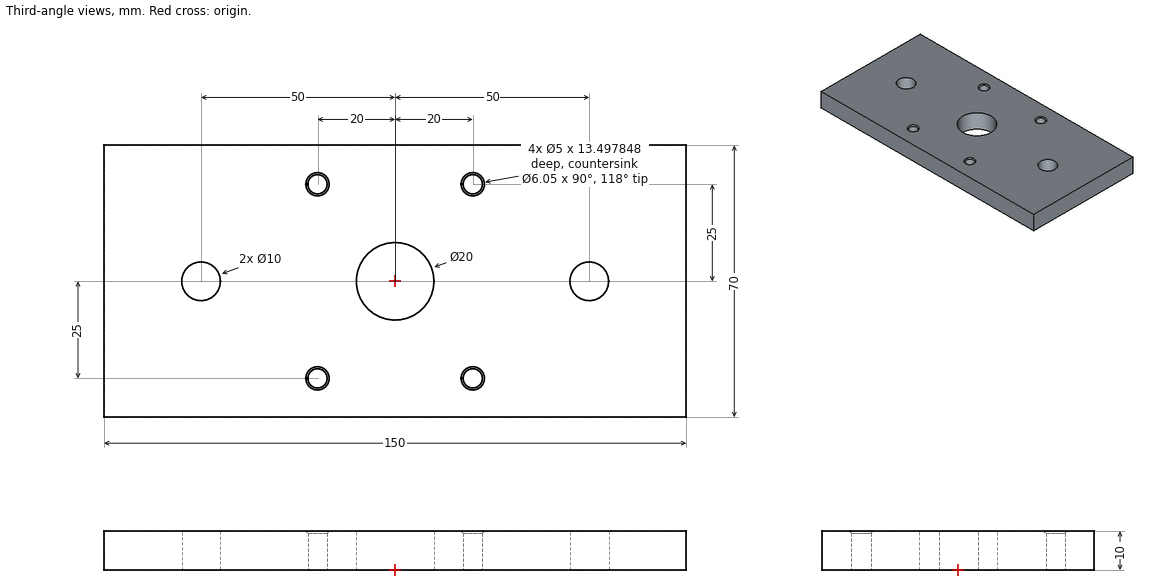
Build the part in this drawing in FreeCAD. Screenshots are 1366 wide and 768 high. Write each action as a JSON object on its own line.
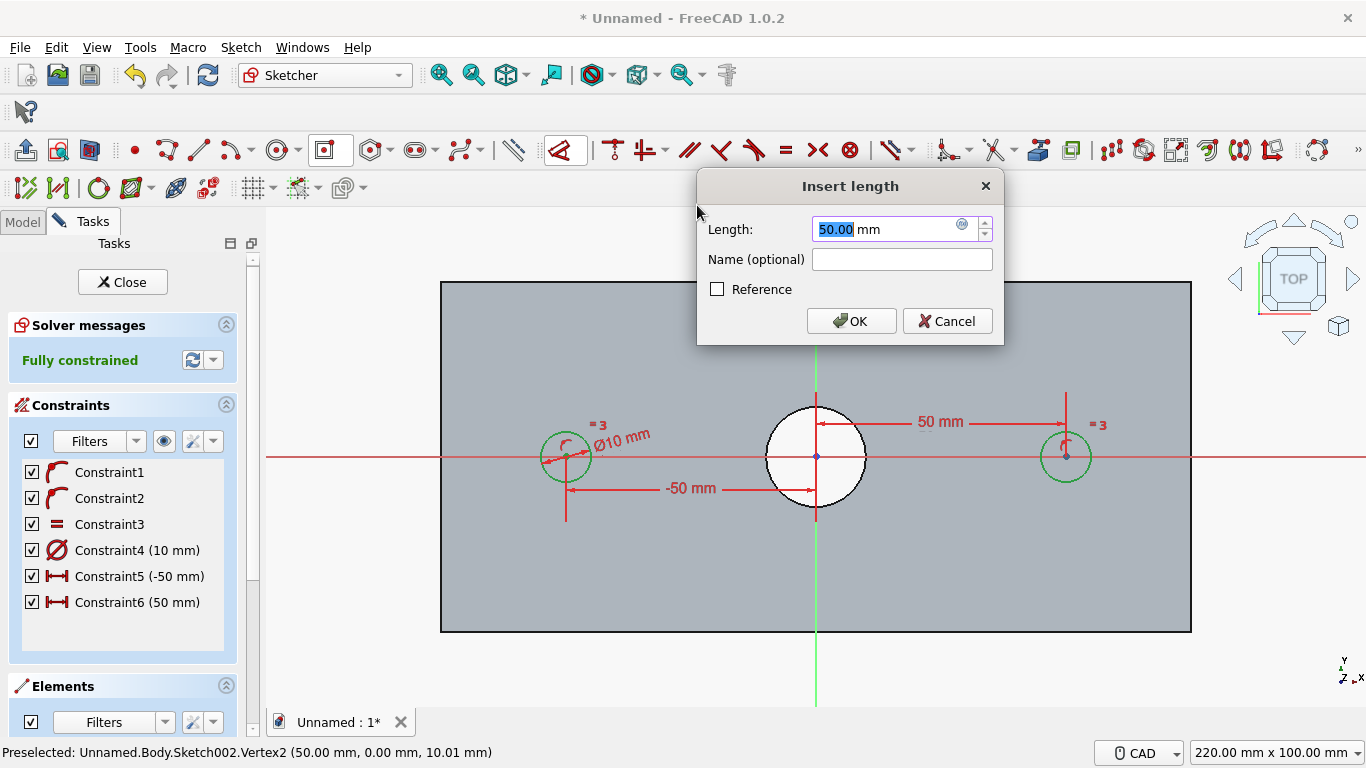
{"action": "type", "text": "50"}
{"action": "key", "text": "Return"}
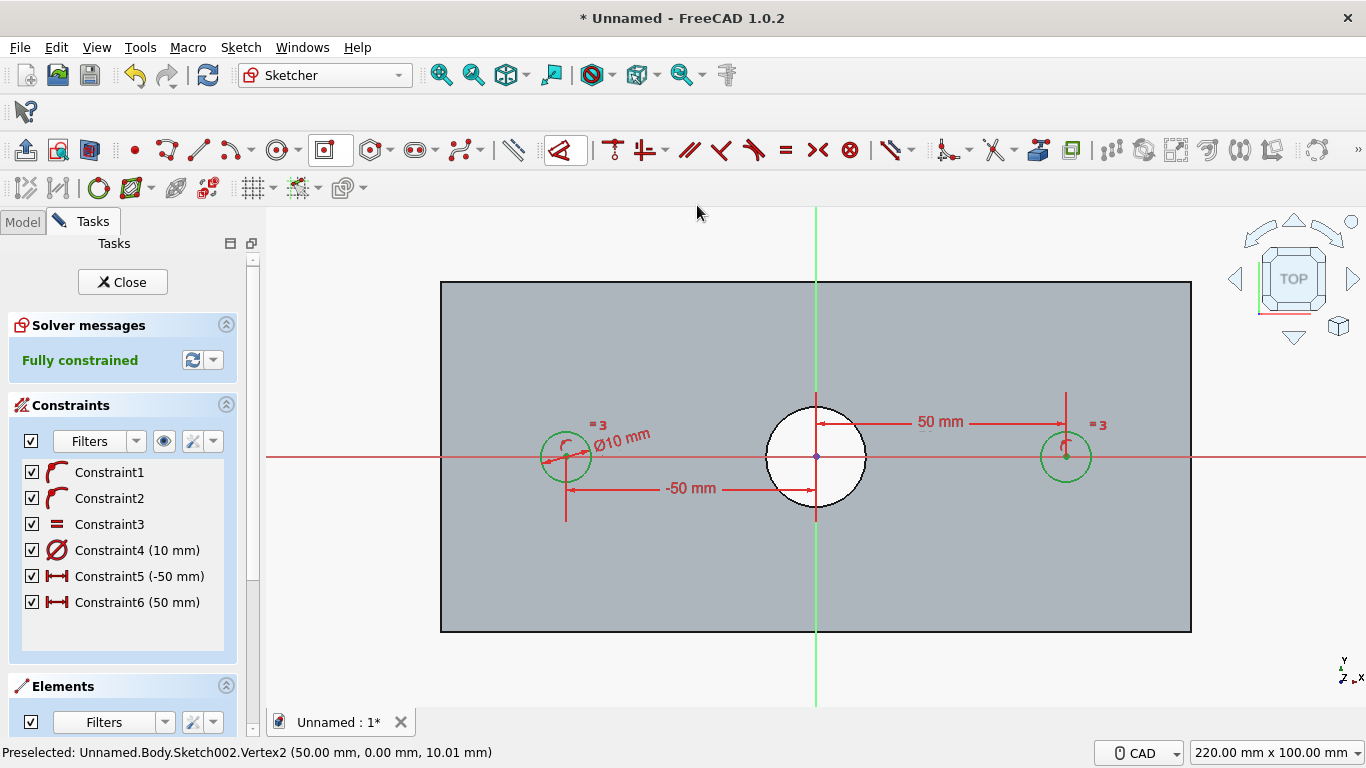
{"action": "left_click", "coordinate": [123, 282]}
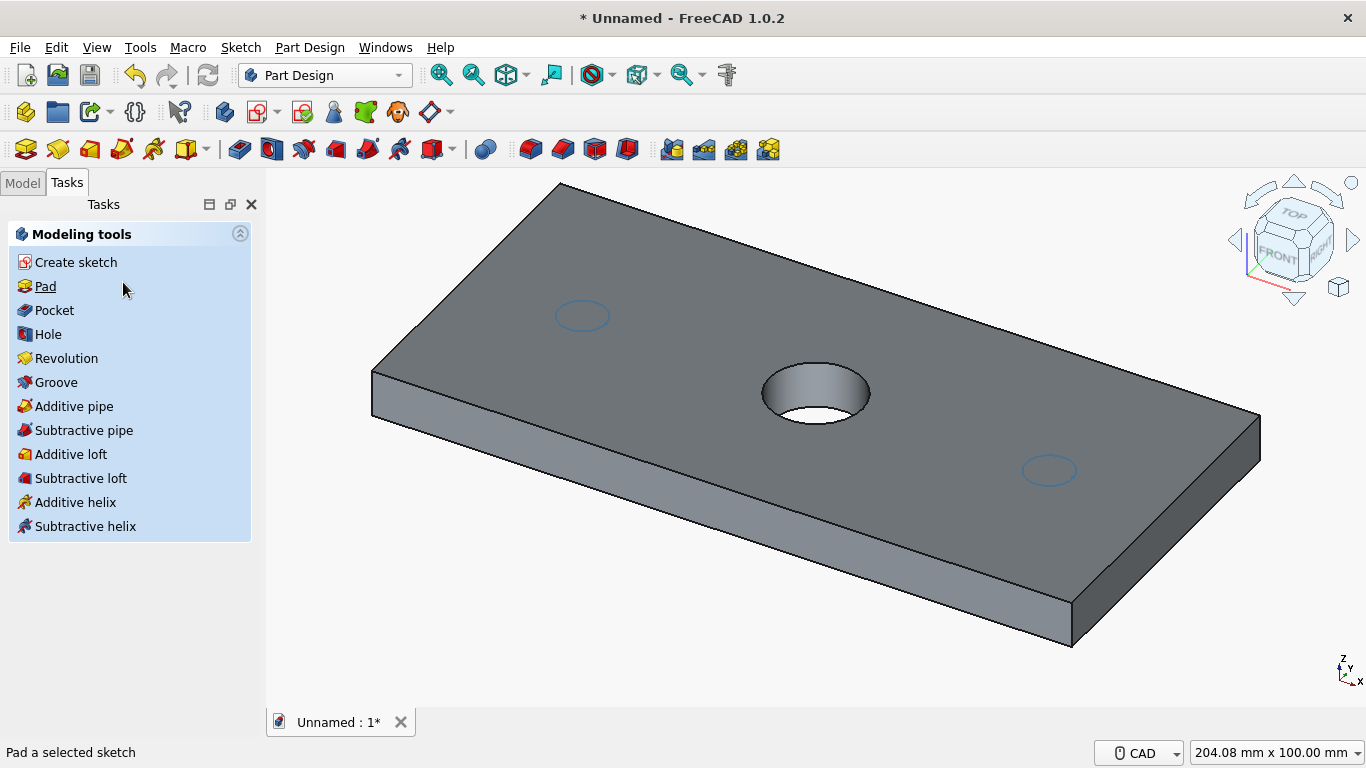
{"action": "left_click", "coordinate": [240, 150]}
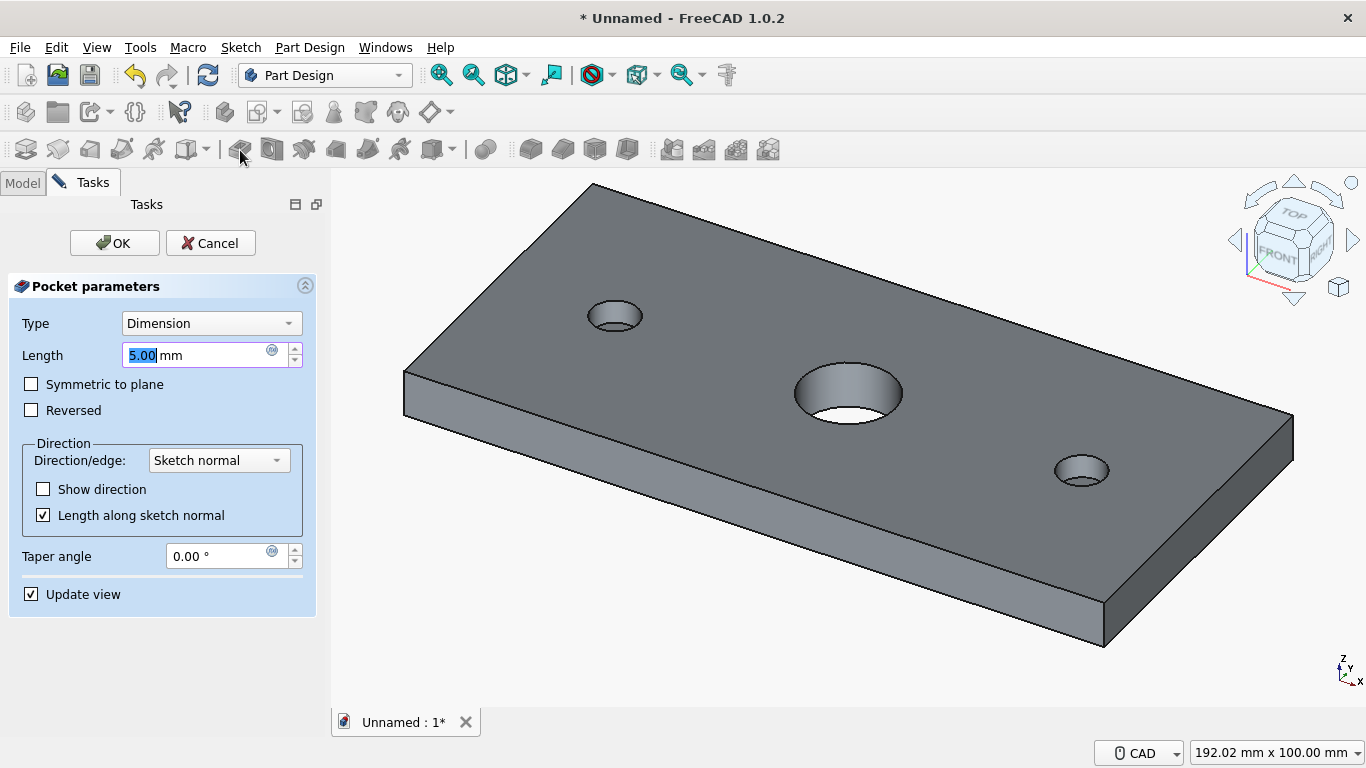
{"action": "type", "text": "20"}
{"action": "key", "text": "Tab"}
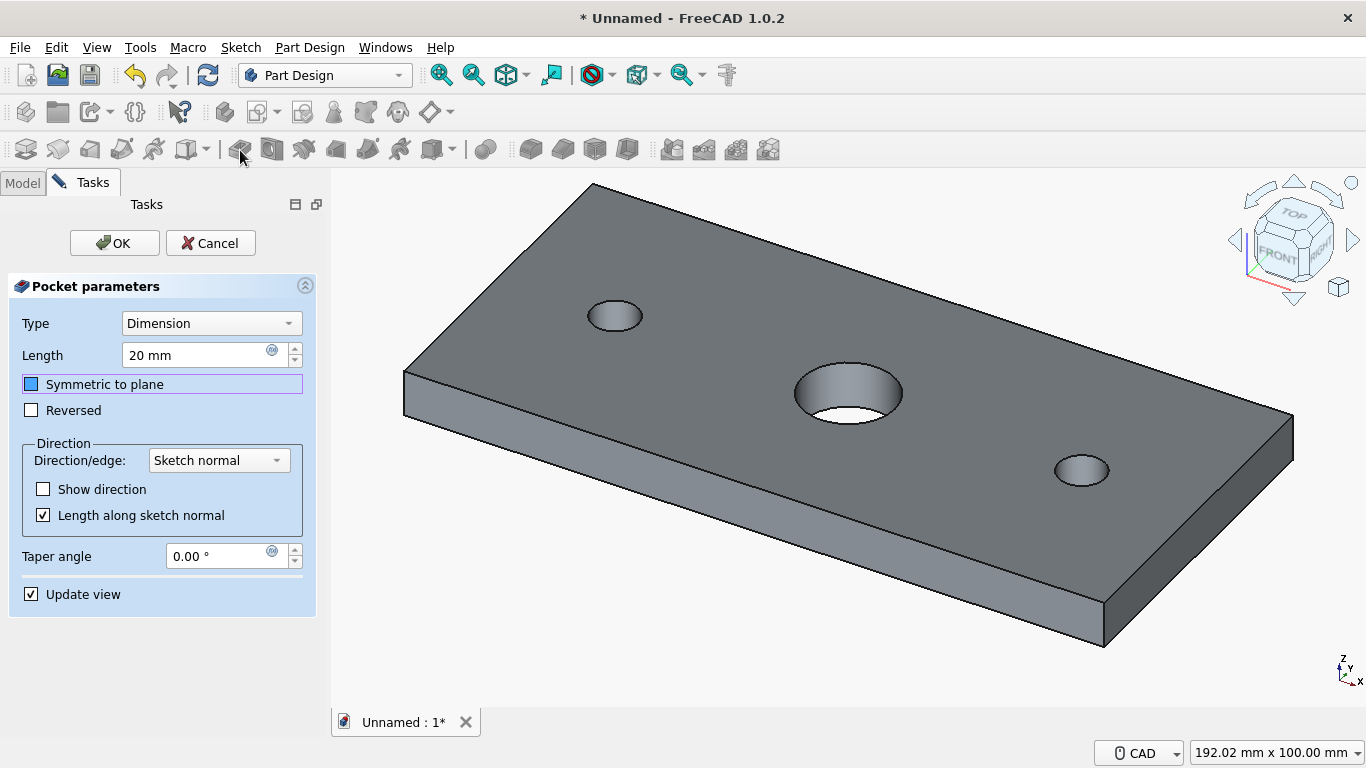
{"action": "left_click", "coordinate": [115, 243]}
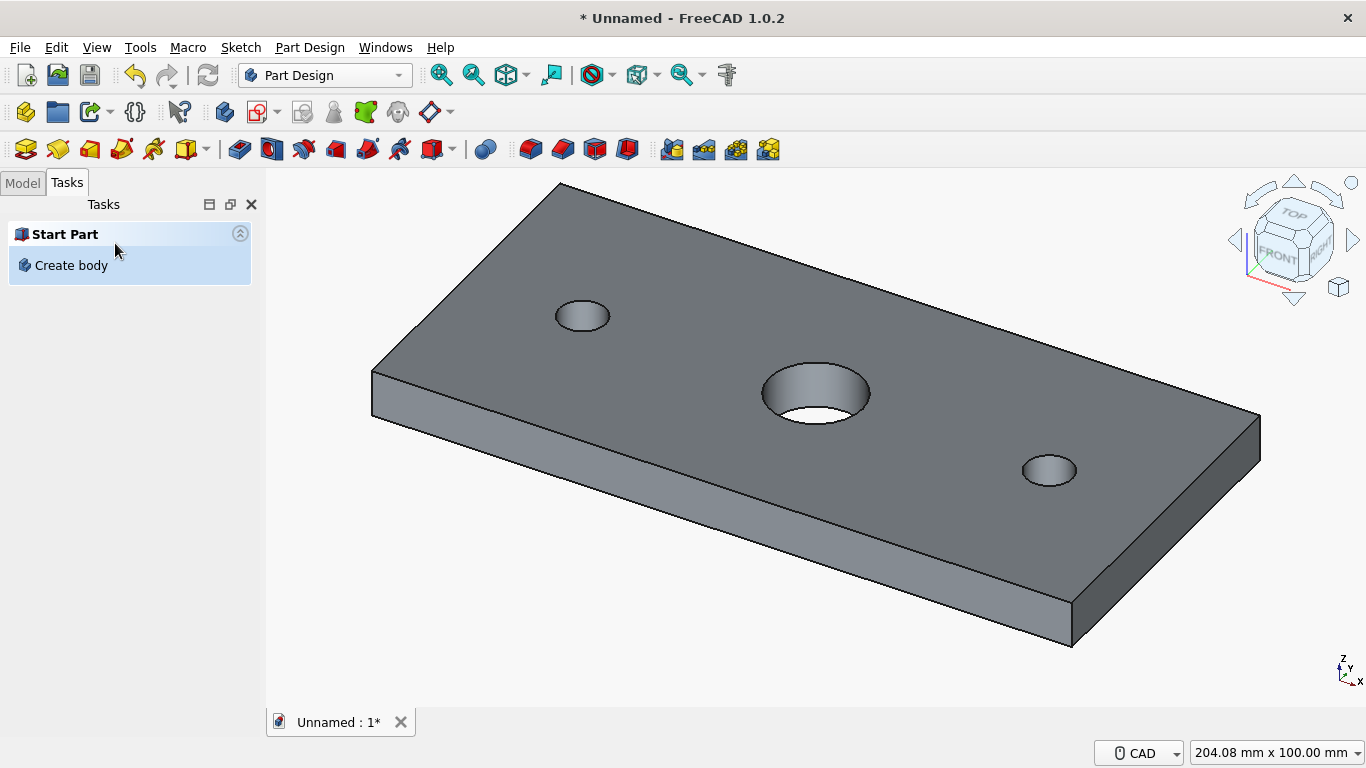
{"action": "left_click", "coordinate": [1070, 405]}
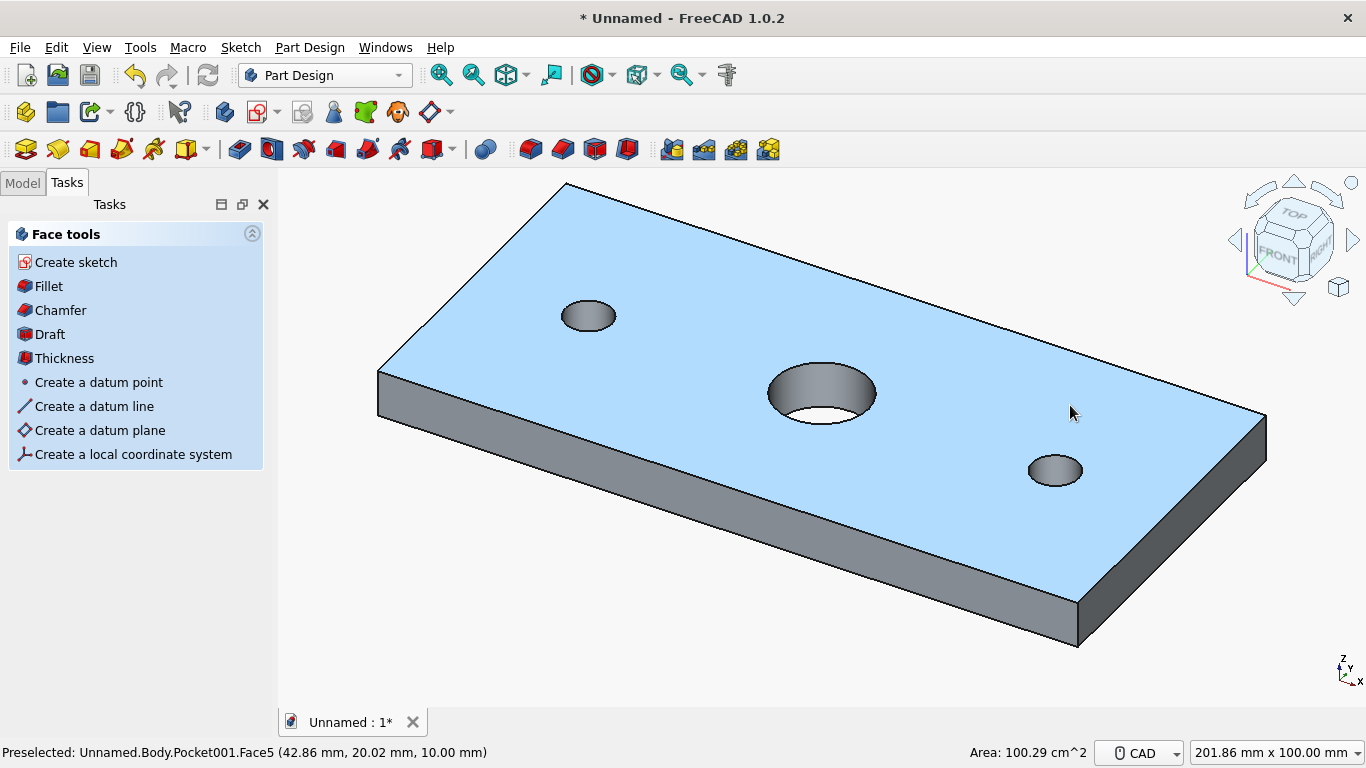
{"action": "left_click", "coordinate": [258, 112]}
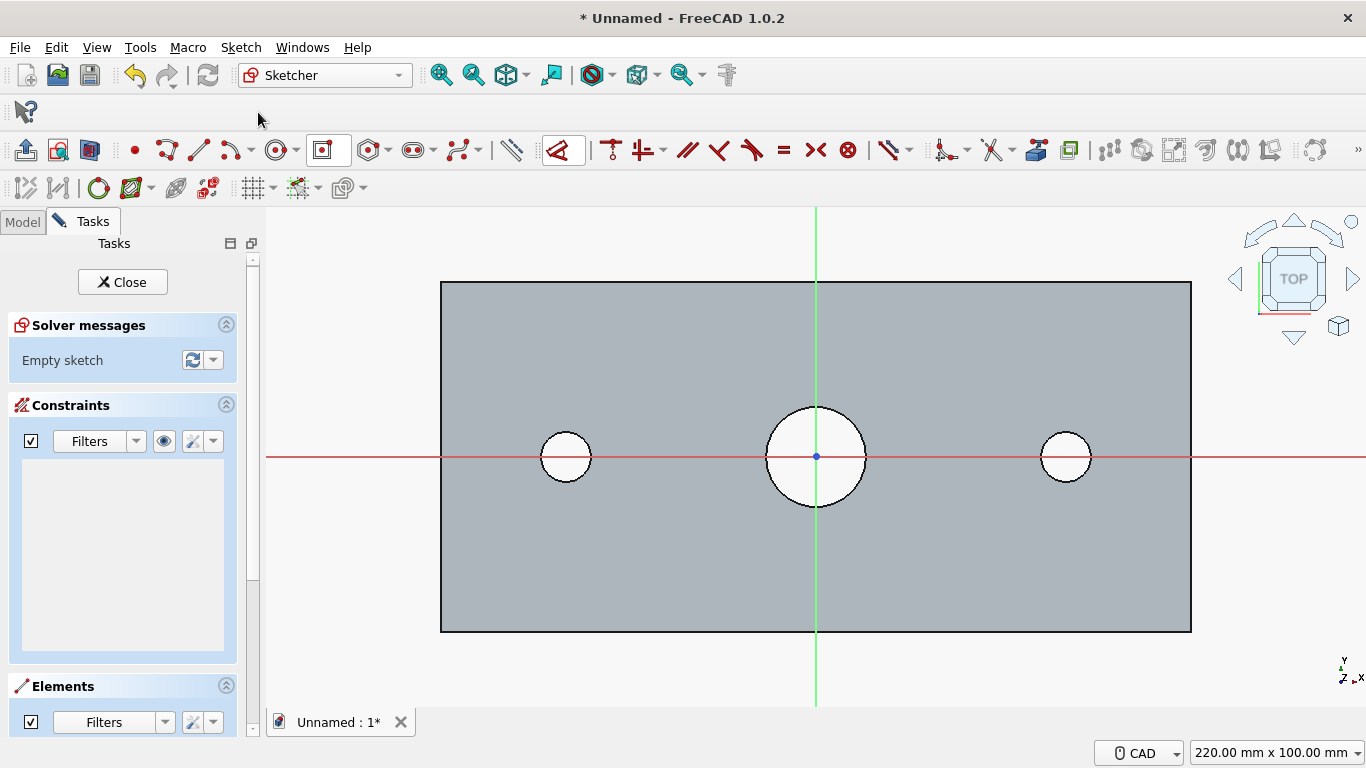
{"action": "left_click", "coordinate": [276, 150]}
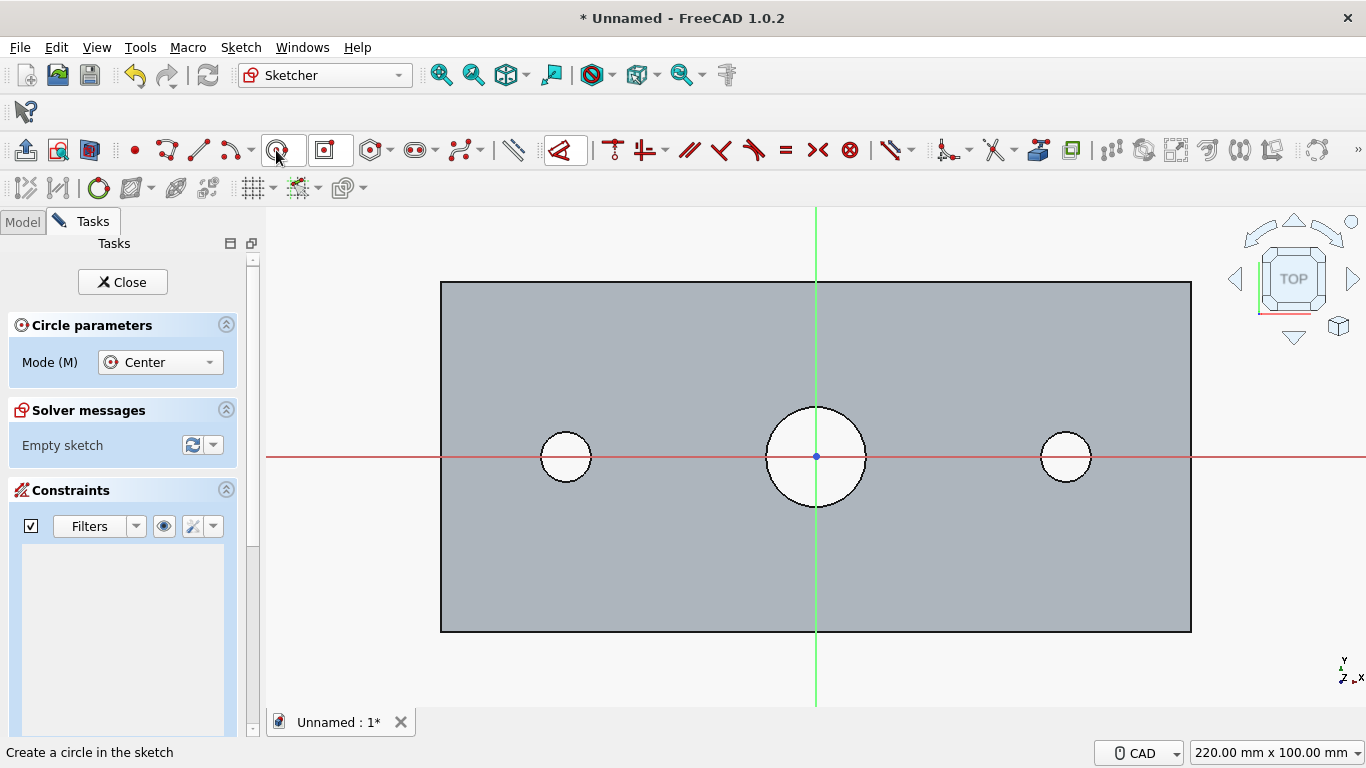
{"action": "scroll", "coordinate": [916, 332], "scroll_direction": "up", "scroll_amount": 3}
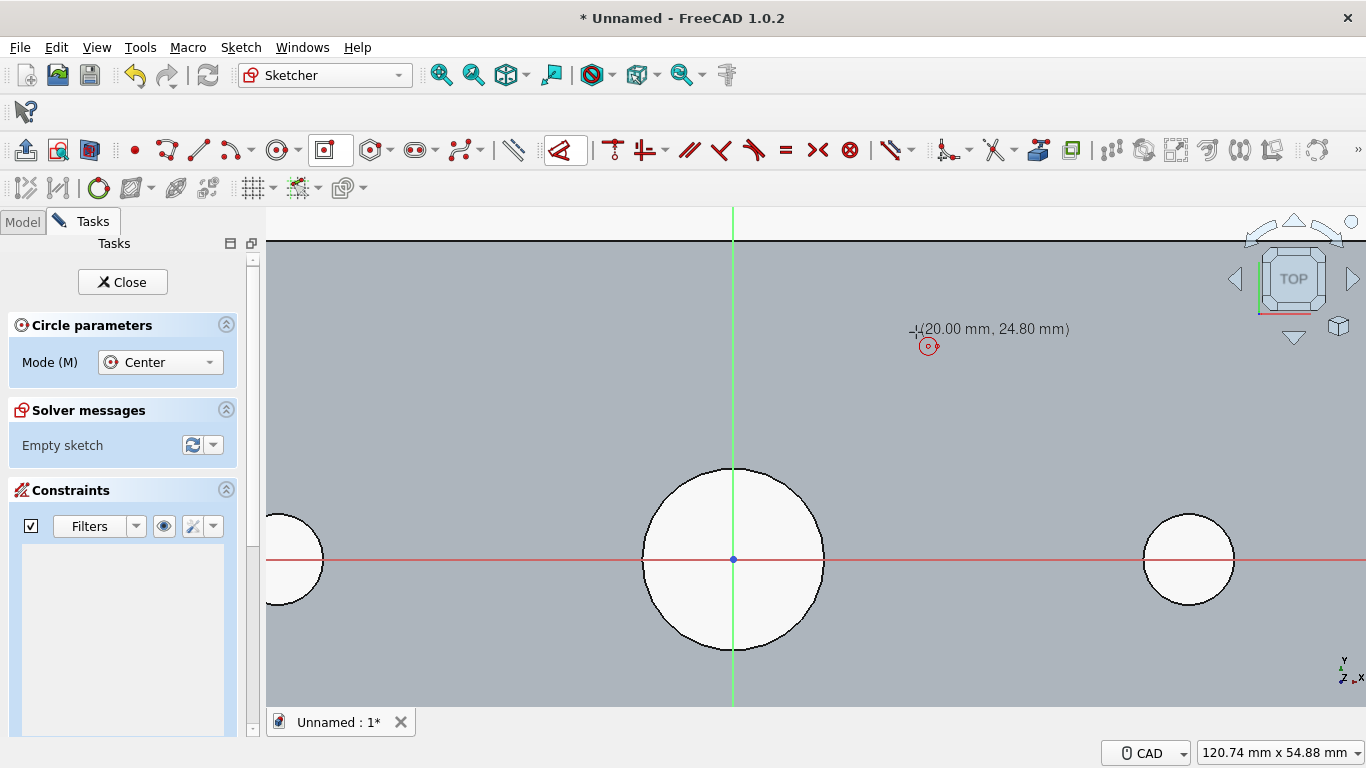
{"action": "left_click", "coordinate": [916, 332]}
{"action": "left_click", "coordinate": [932, 316]}